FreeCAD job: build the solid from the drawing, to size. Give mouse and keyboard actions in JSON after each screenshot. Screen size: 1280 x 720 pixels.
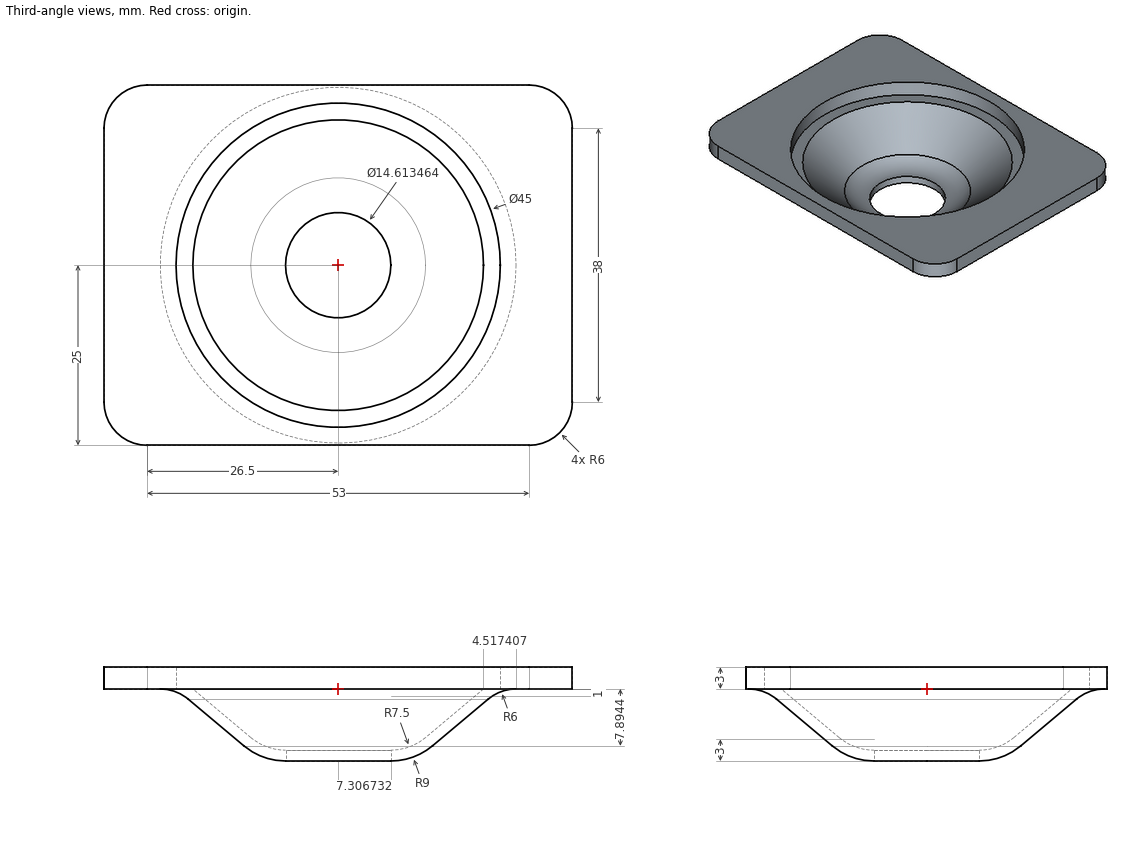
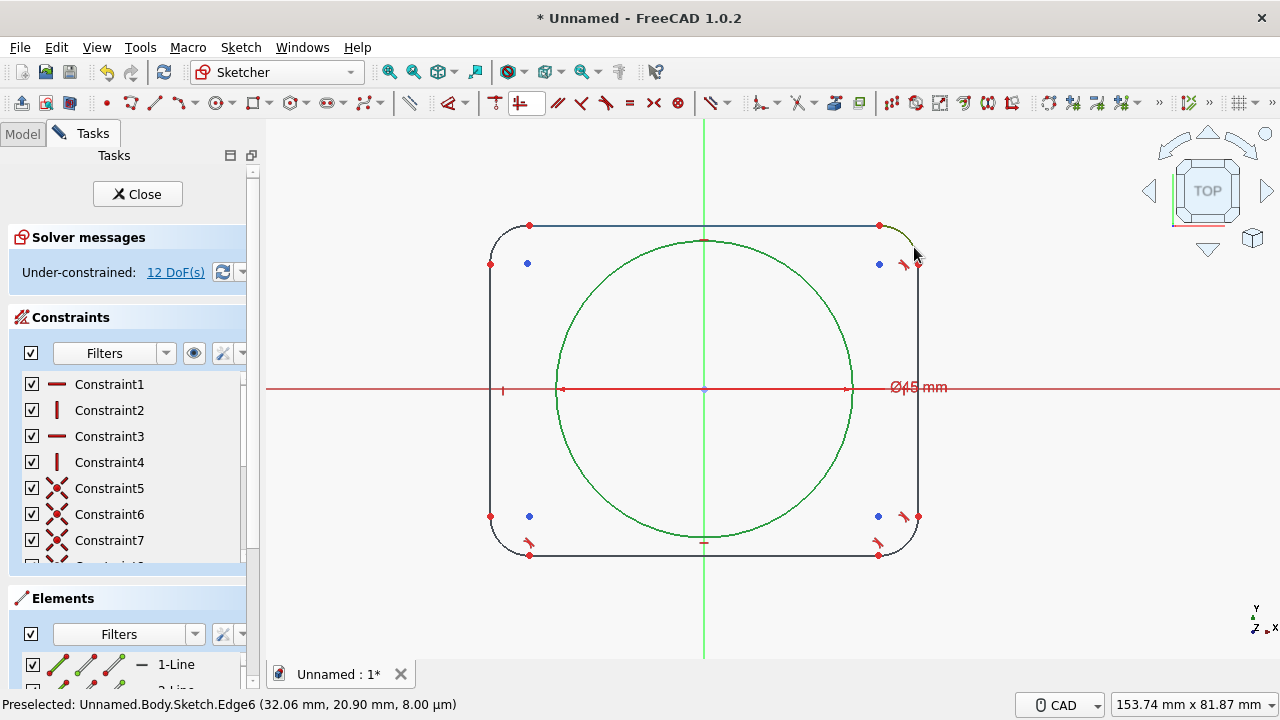
{"action": "key", "text": "t"}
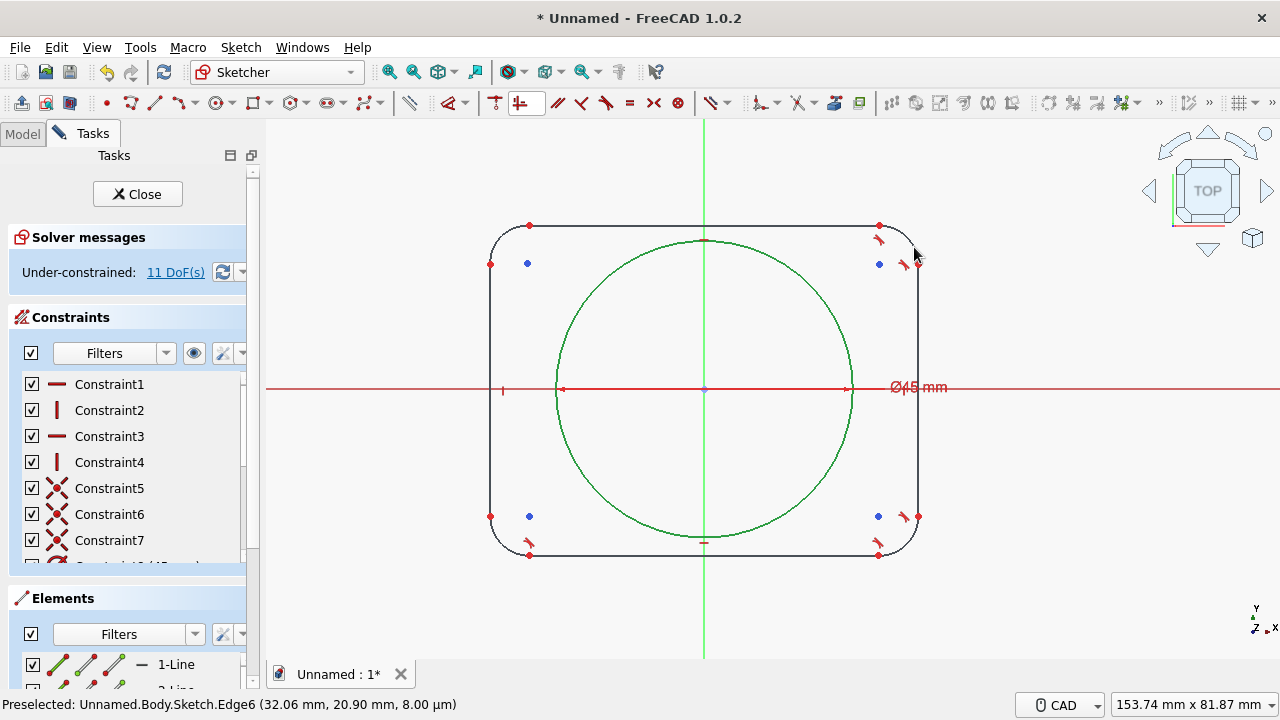
{"action": "left_click", "coordinate": [774, 226]}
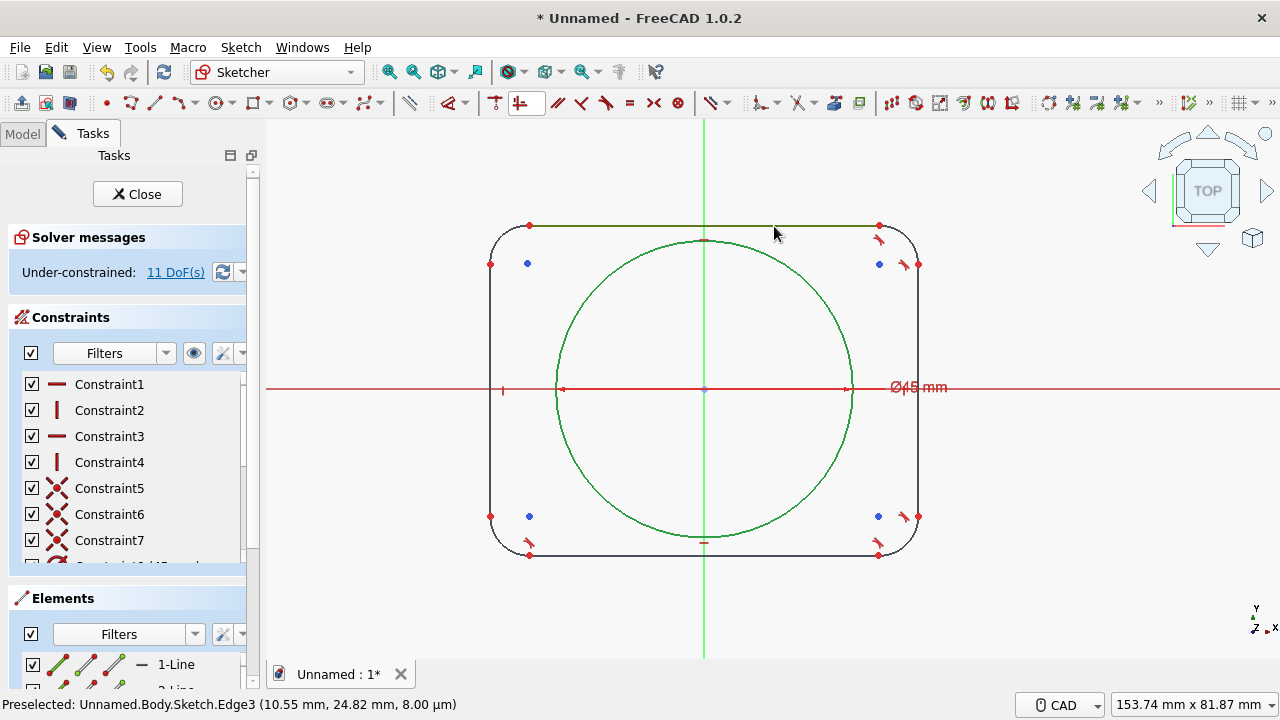
{"action": "left_click", "coordinate": [512, 229]}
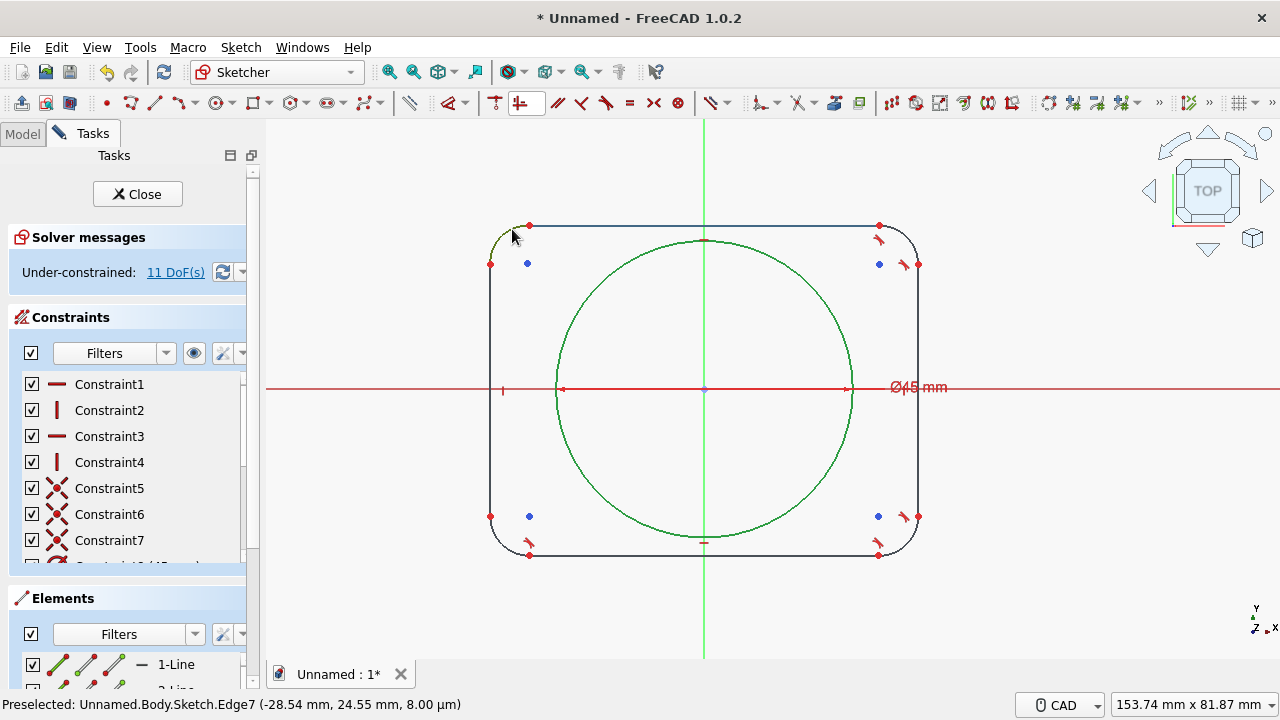
{"action": "left_click", "coordinate": [606, 104]}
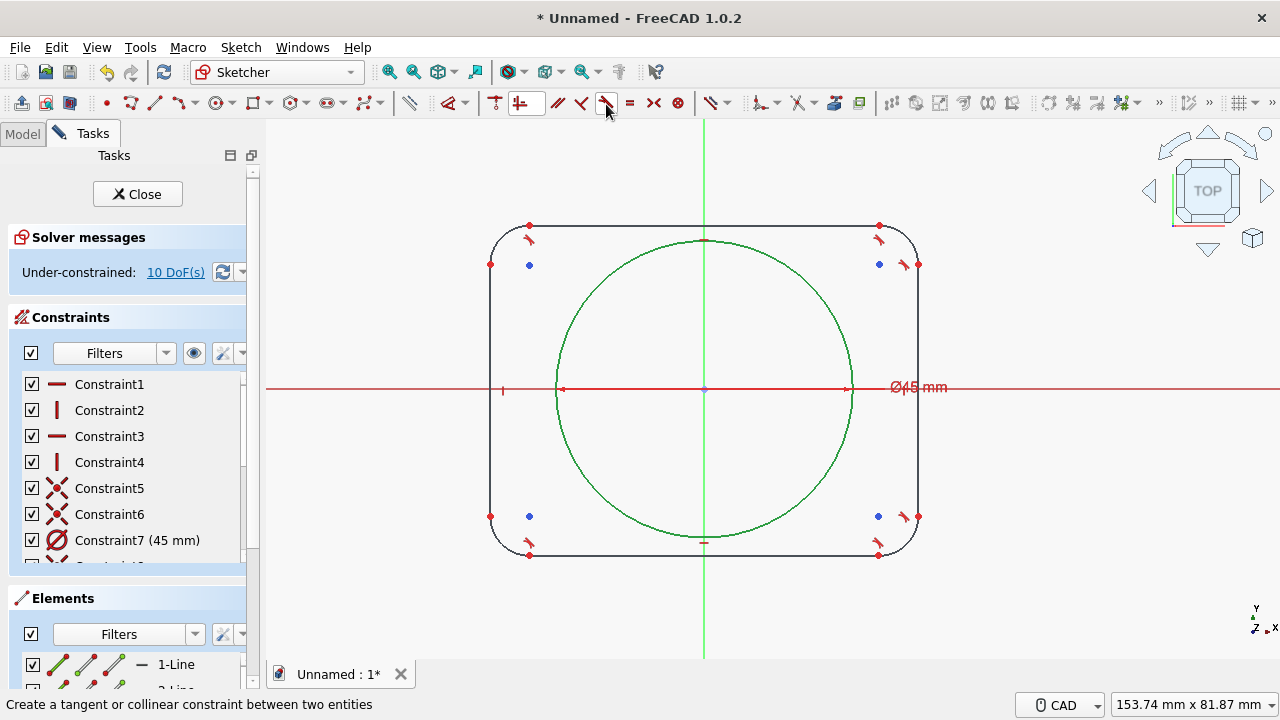
{"action": "left_click", "coordinate": [490, 340]}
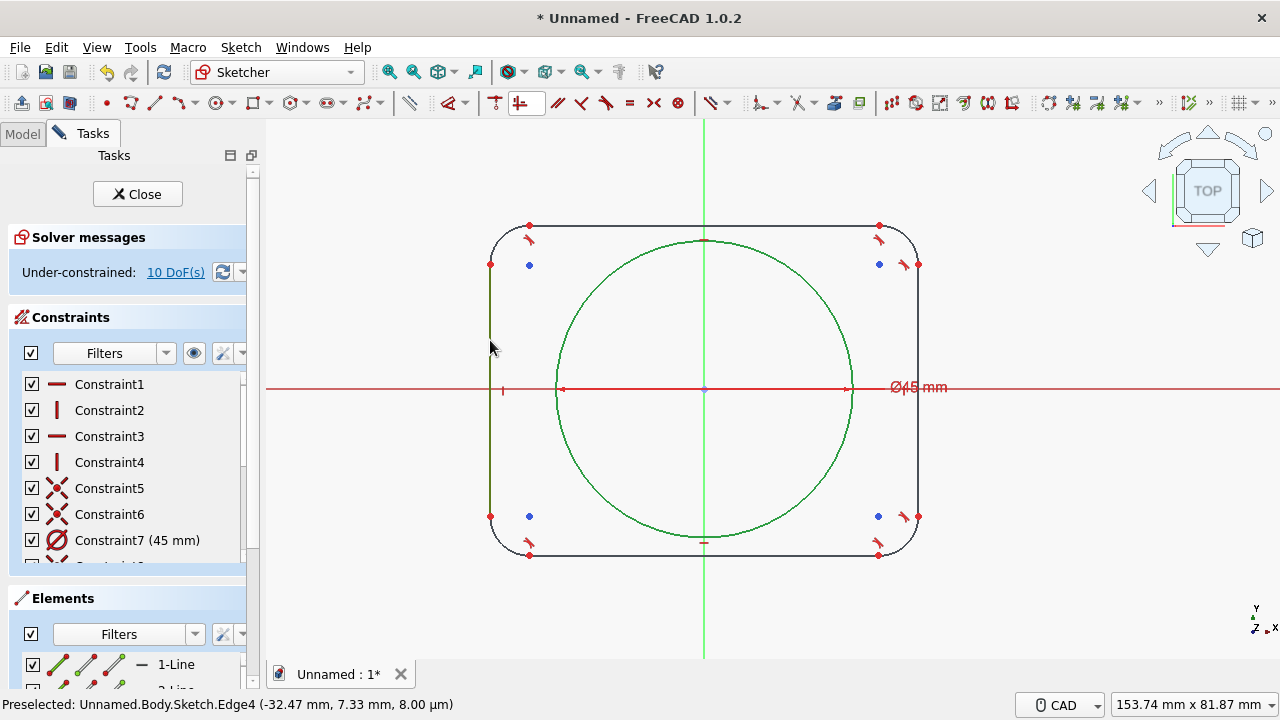
{"action": "left_click", "coordinate": [512, 230]}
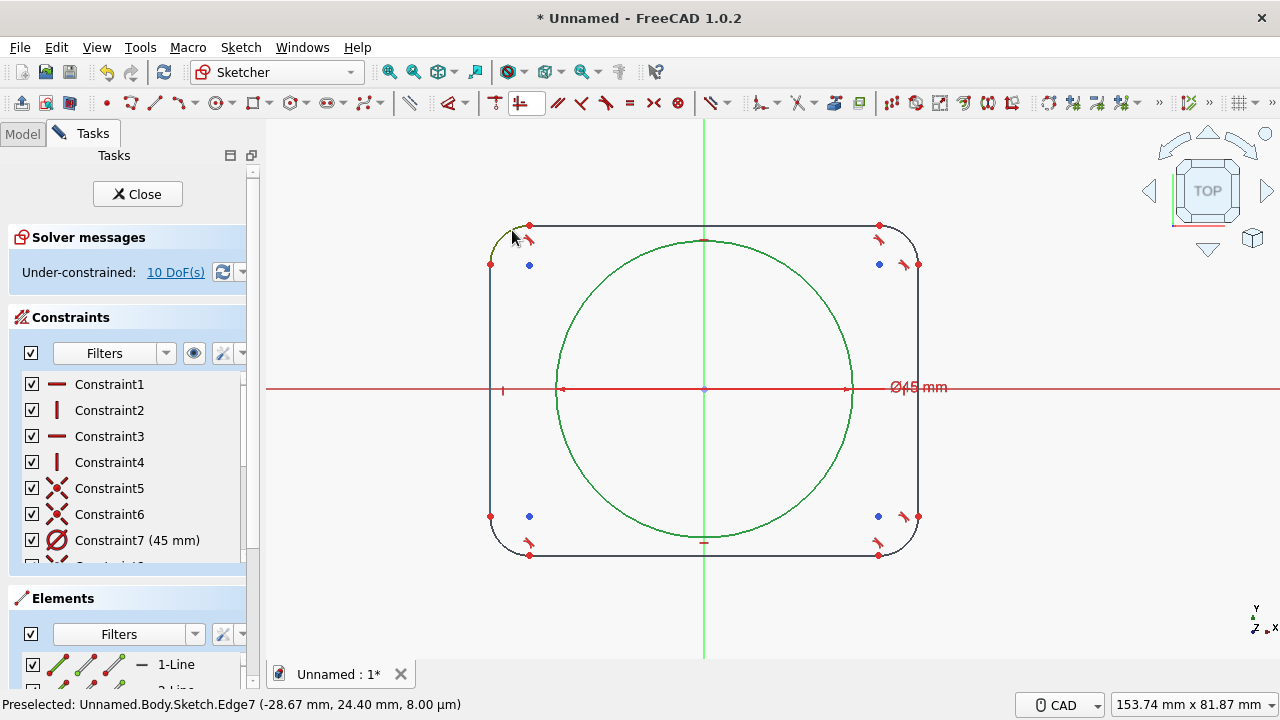
{"action": "key", "text": "t"}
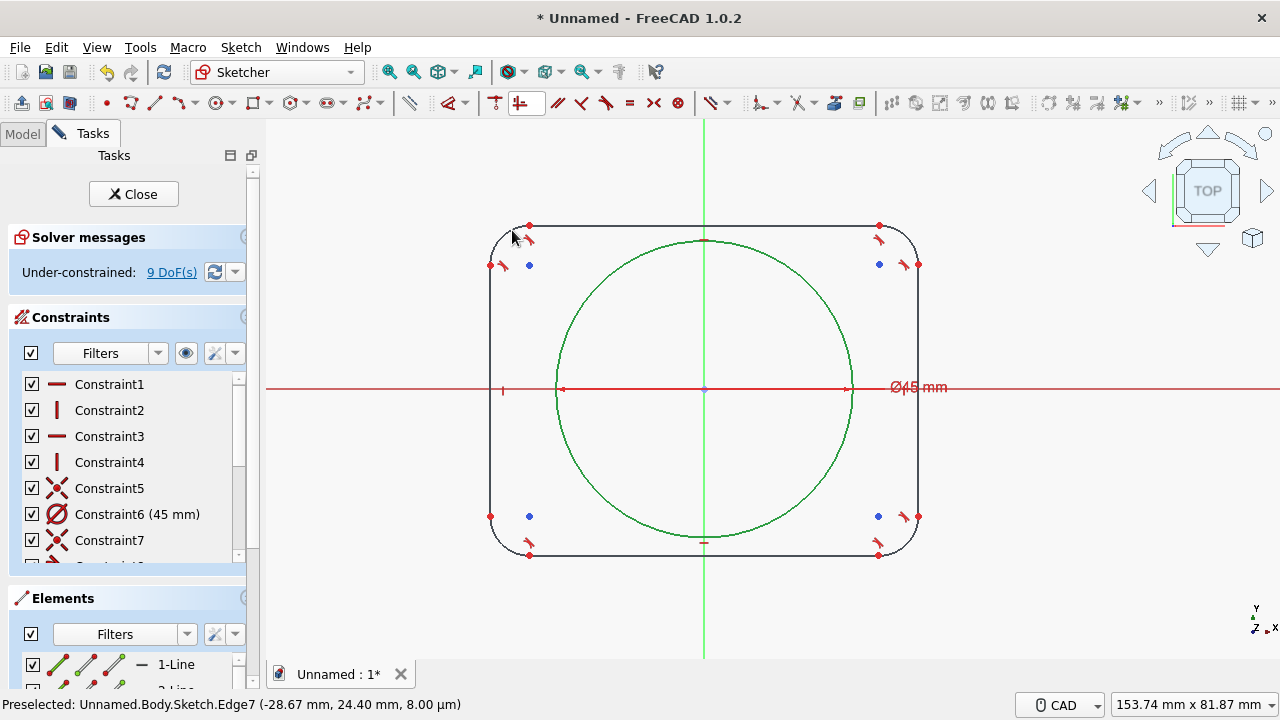
{"action": "left_click", "coordinate": [490, 340]}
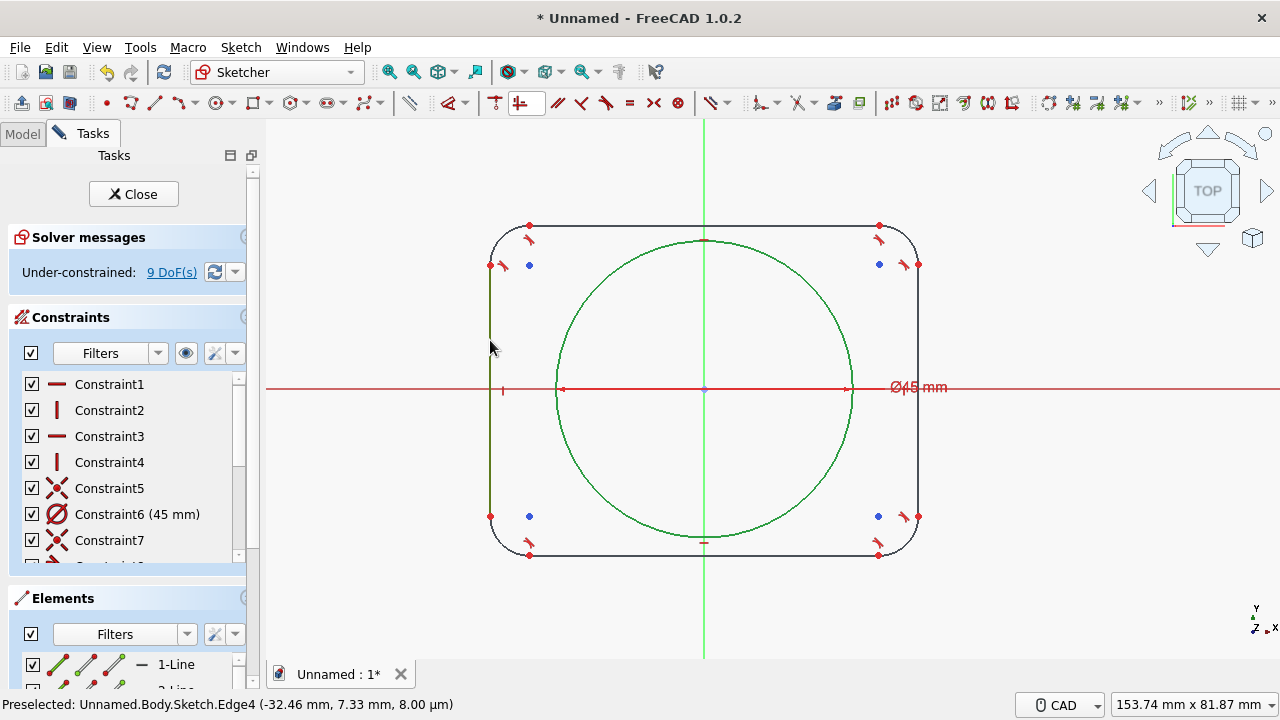
{"action": "left_click", "coordinate": [495, 534]}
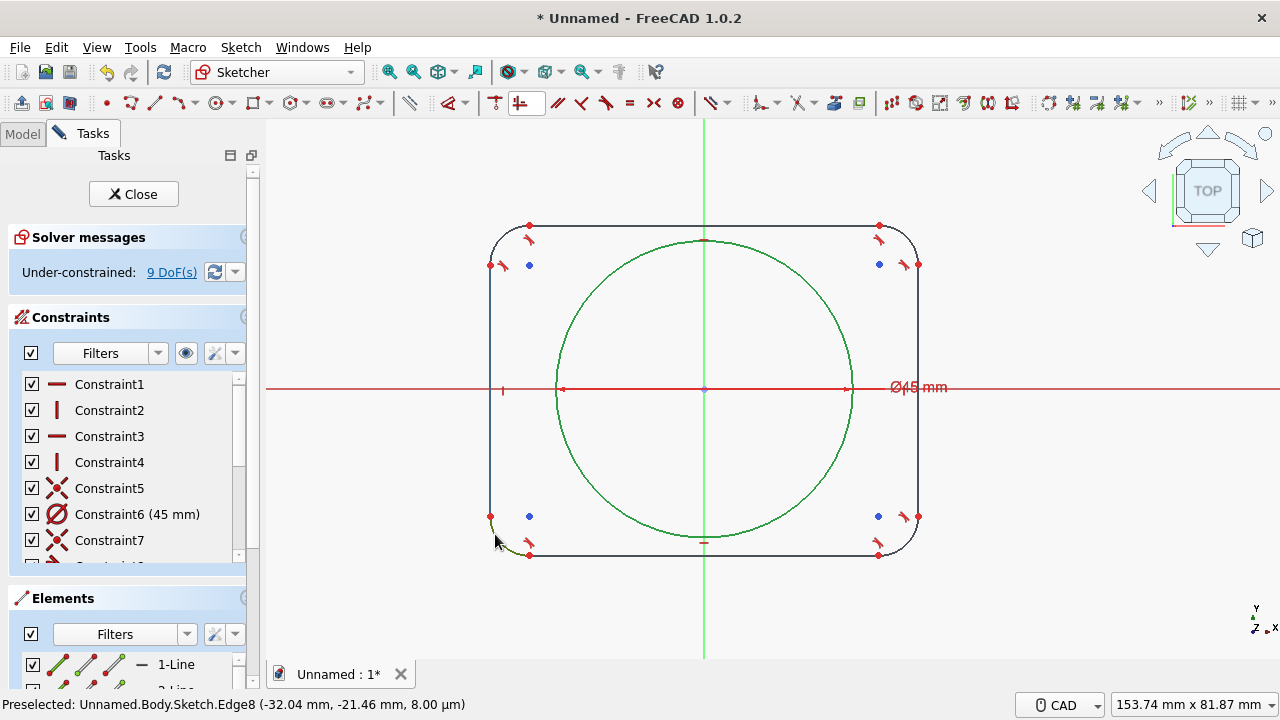
{"action": "key", "text": "t"}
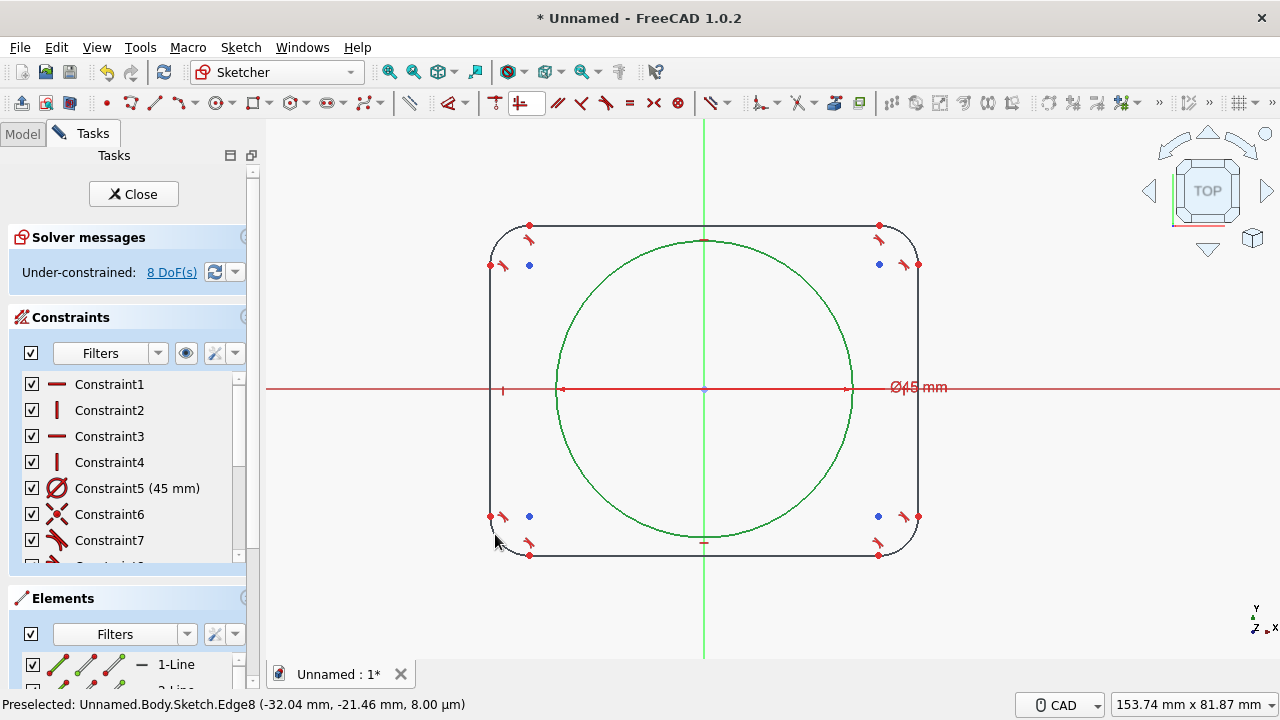
{"action": "left_click", "coordinate": [897, 552]}